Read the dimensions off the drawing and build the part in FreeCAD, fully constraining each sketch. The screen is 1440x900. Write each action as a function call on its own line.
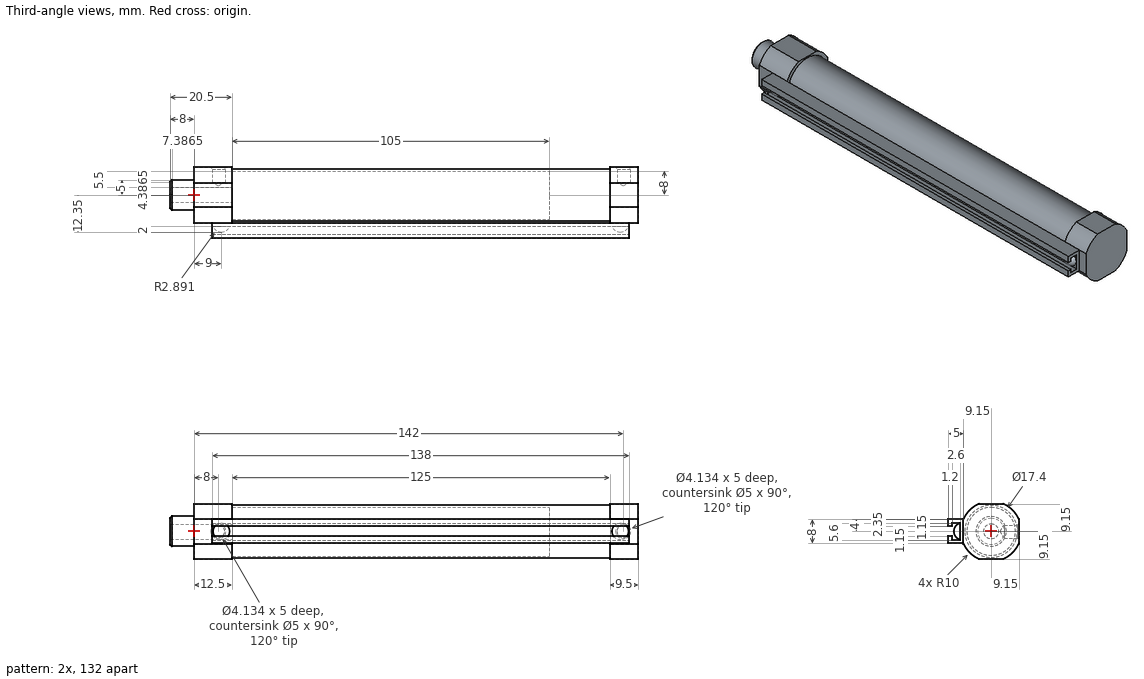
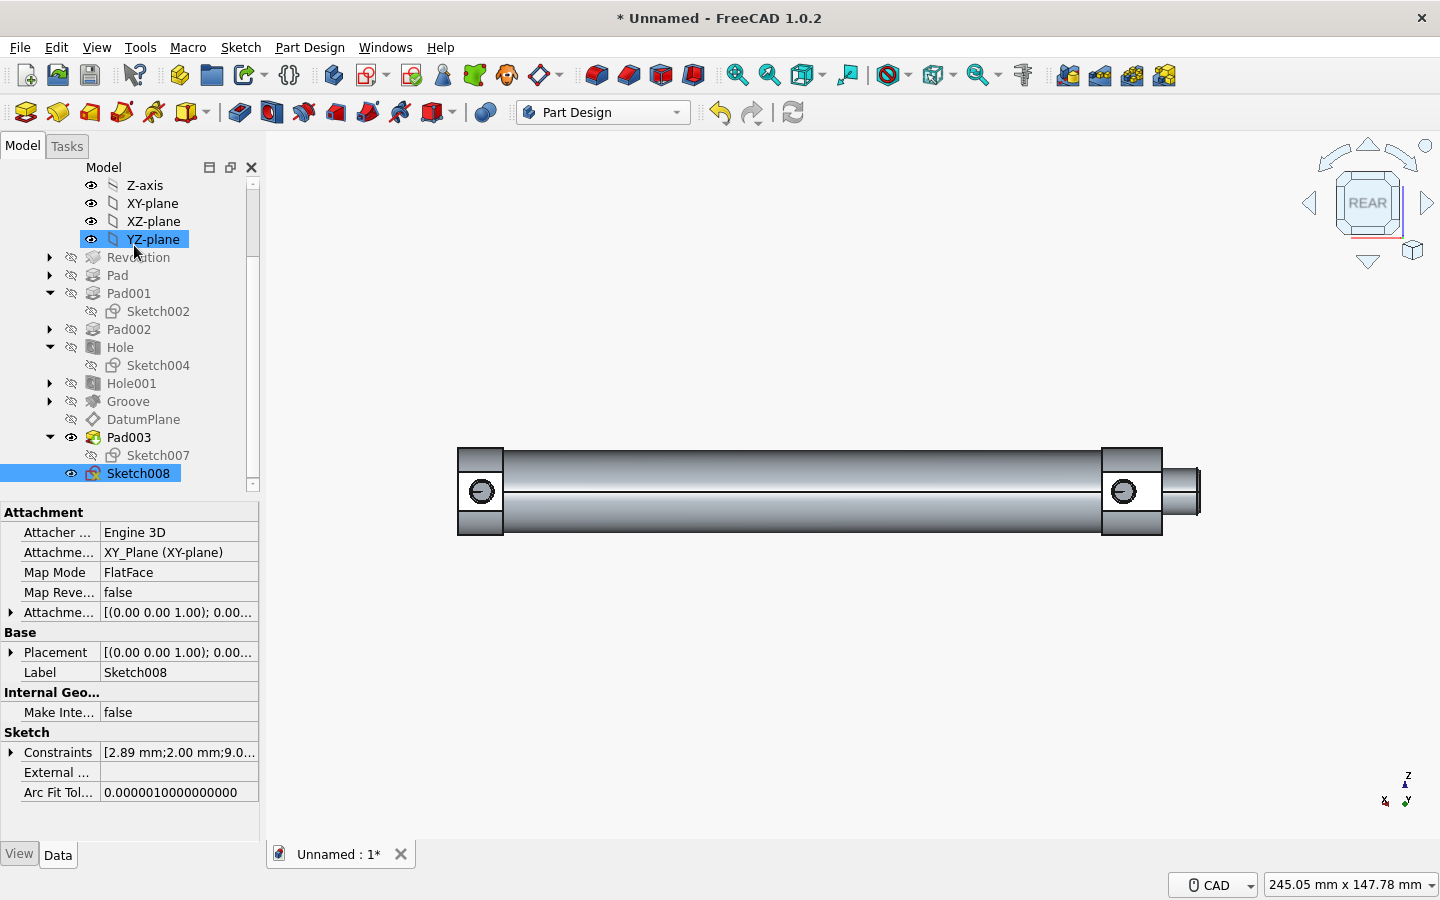
click(58, 112)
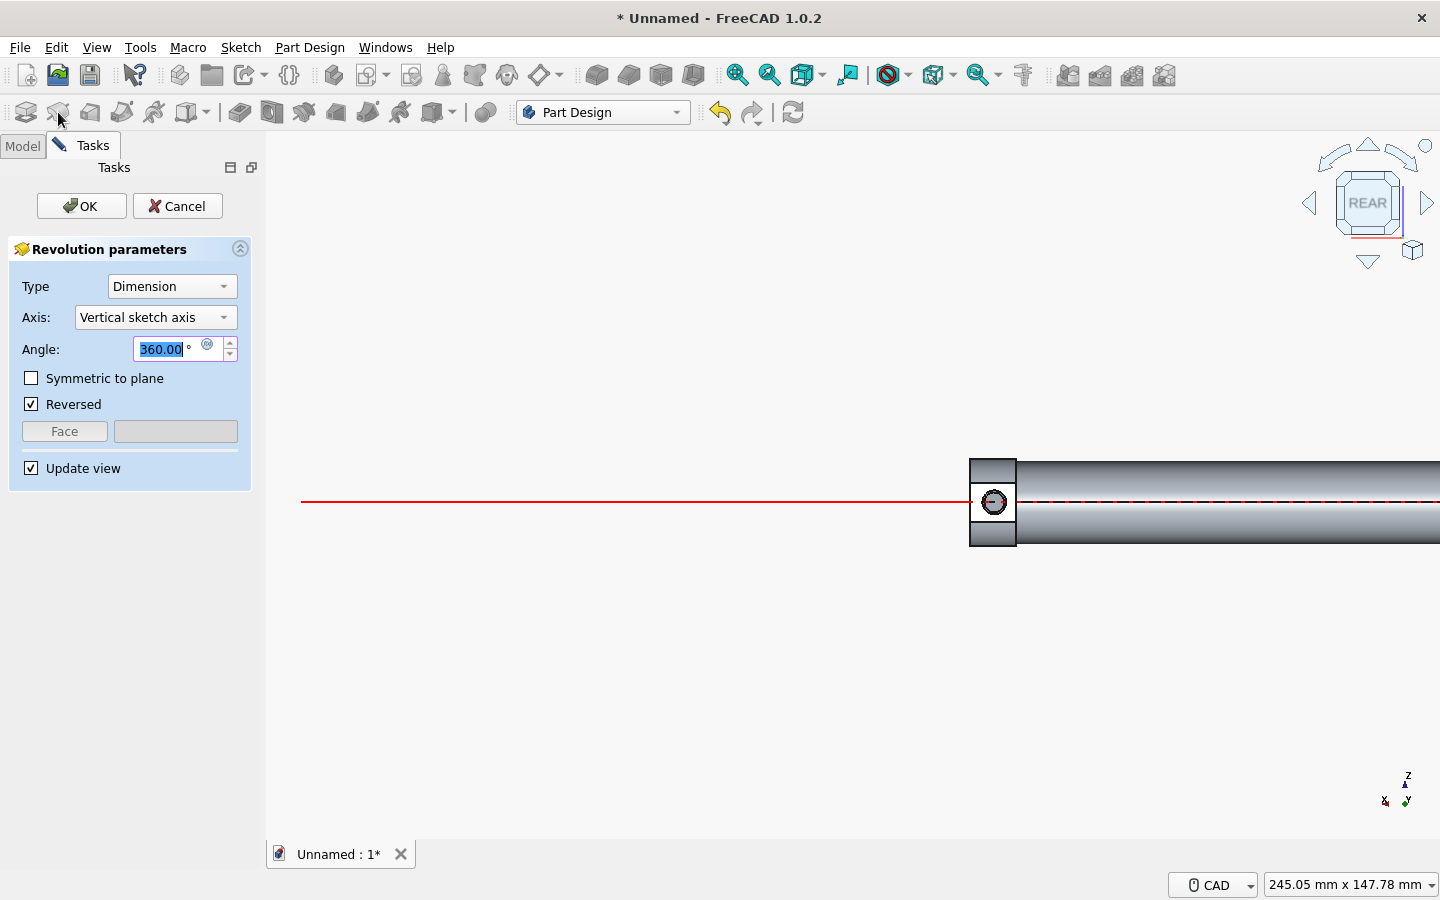
click(156, 318)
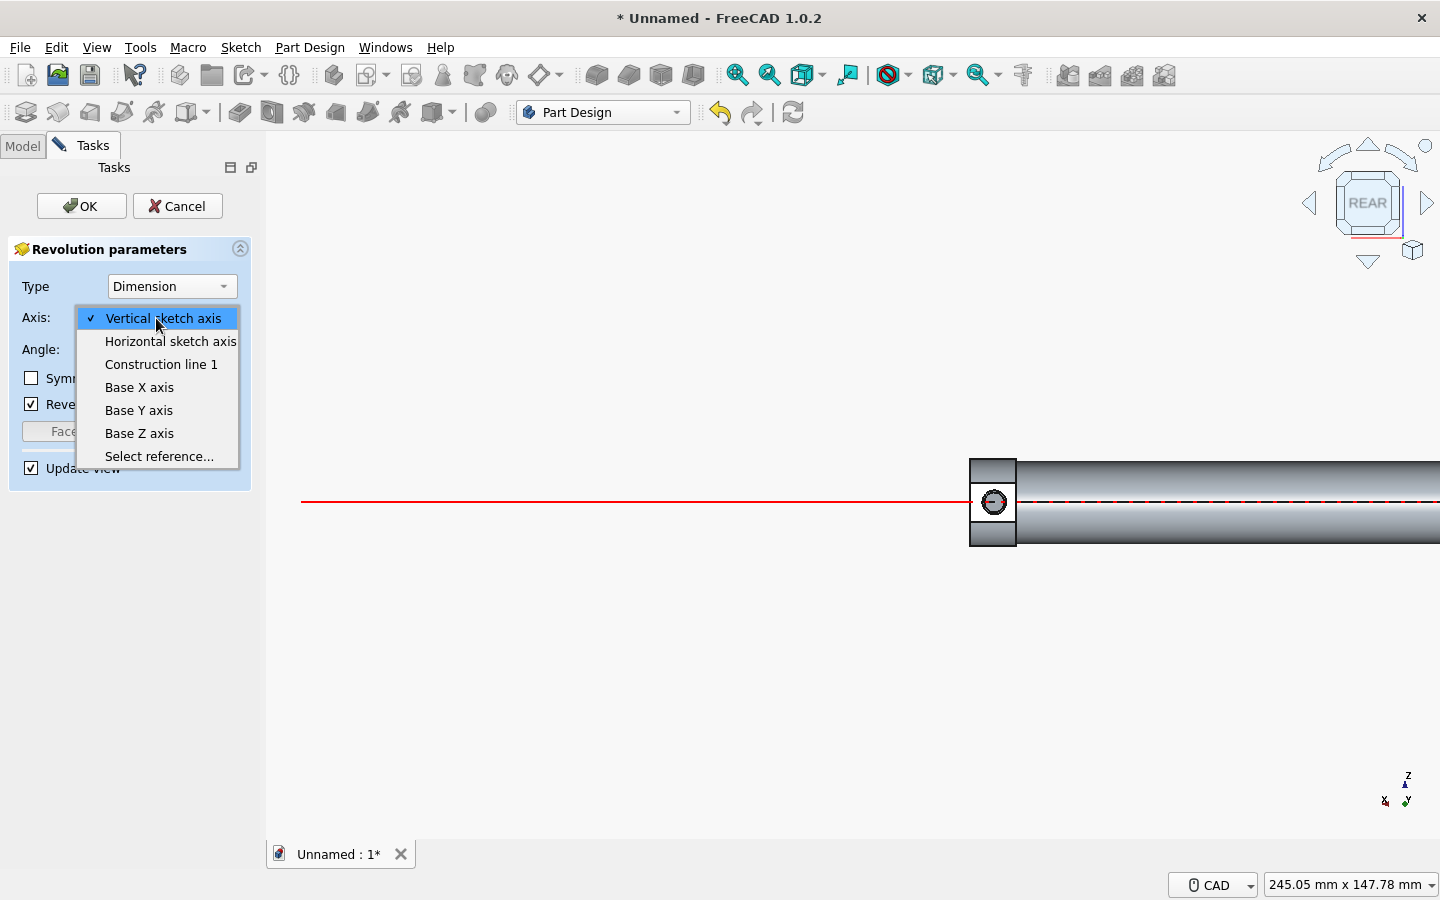
click(156, 364)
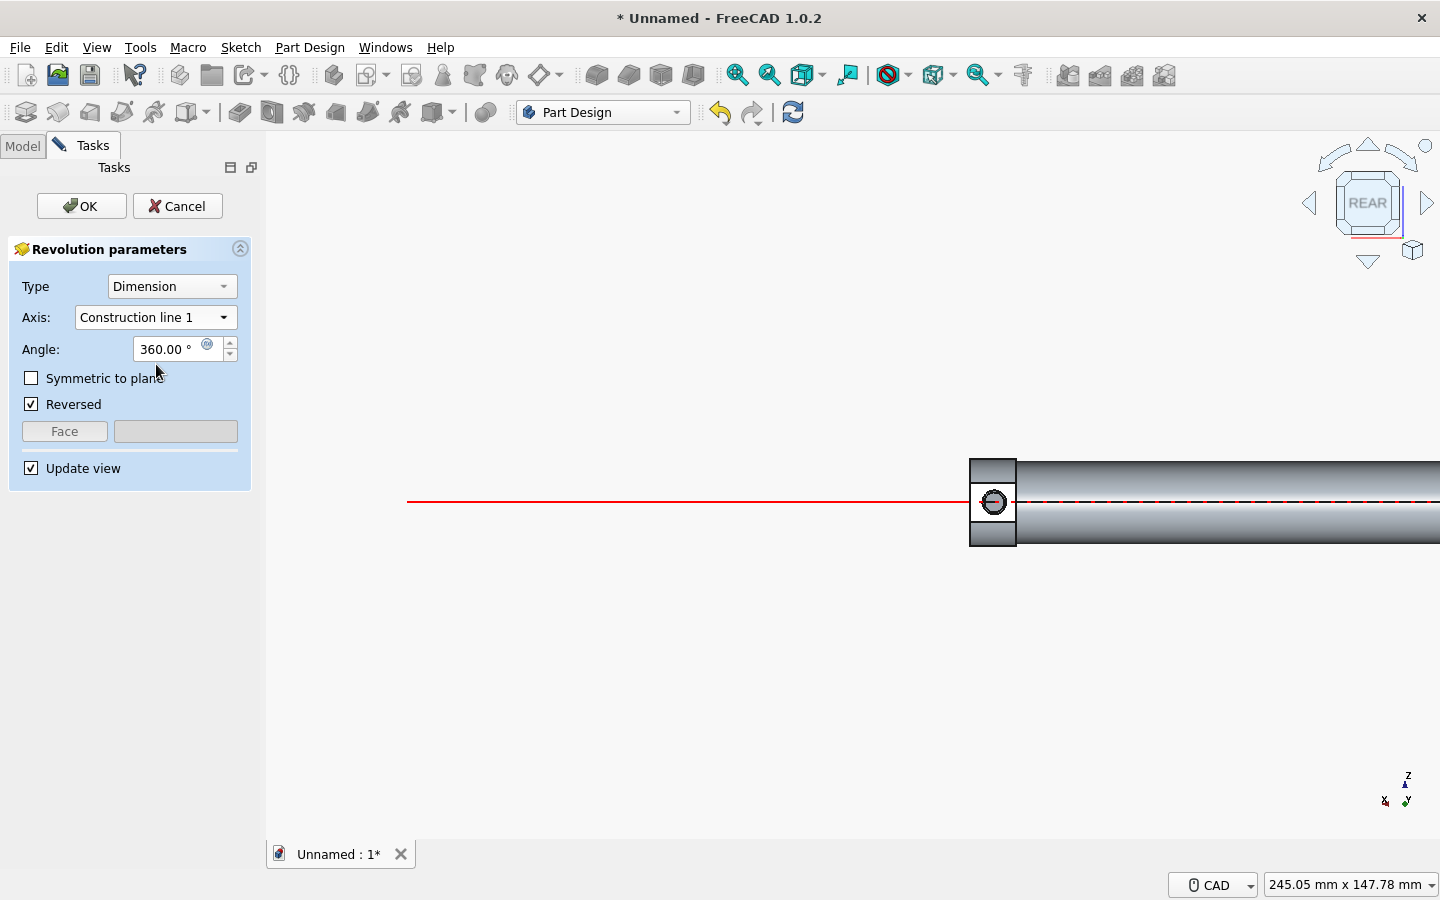
click(82, 206)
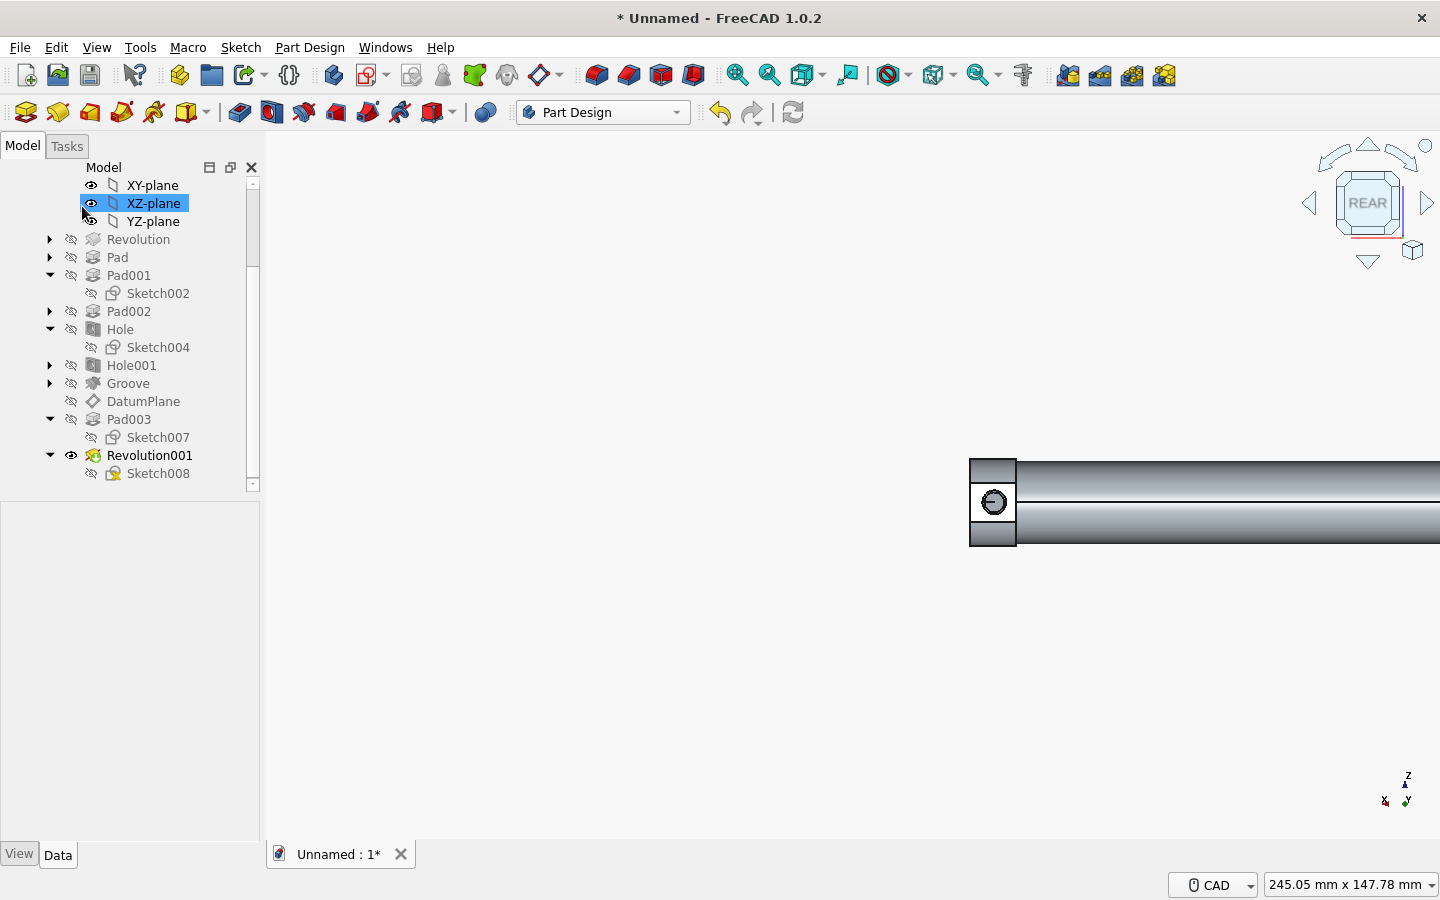
click(738, 76)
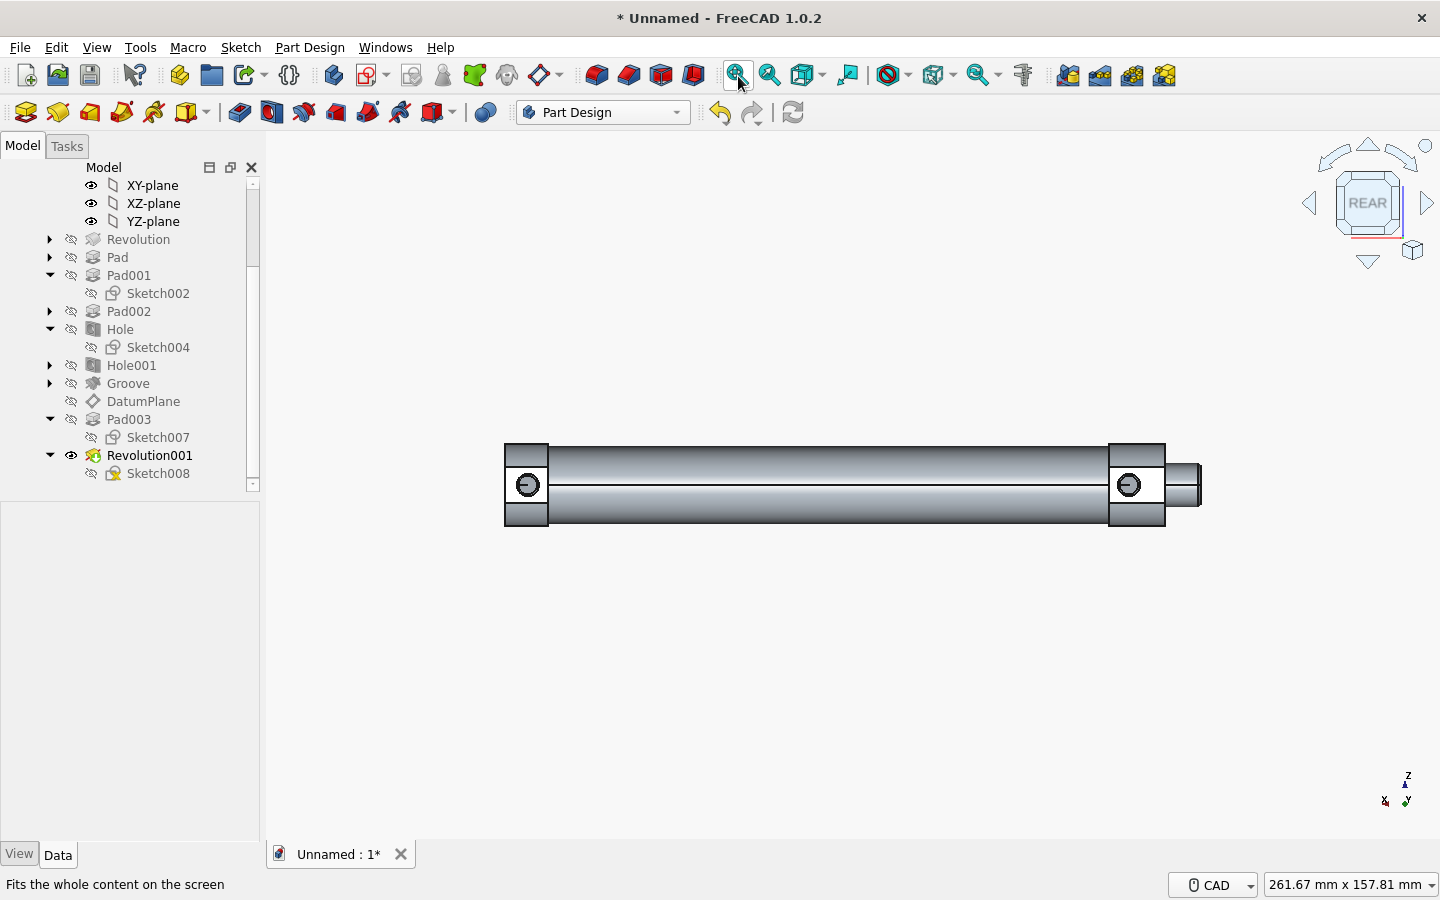
click(116, 455)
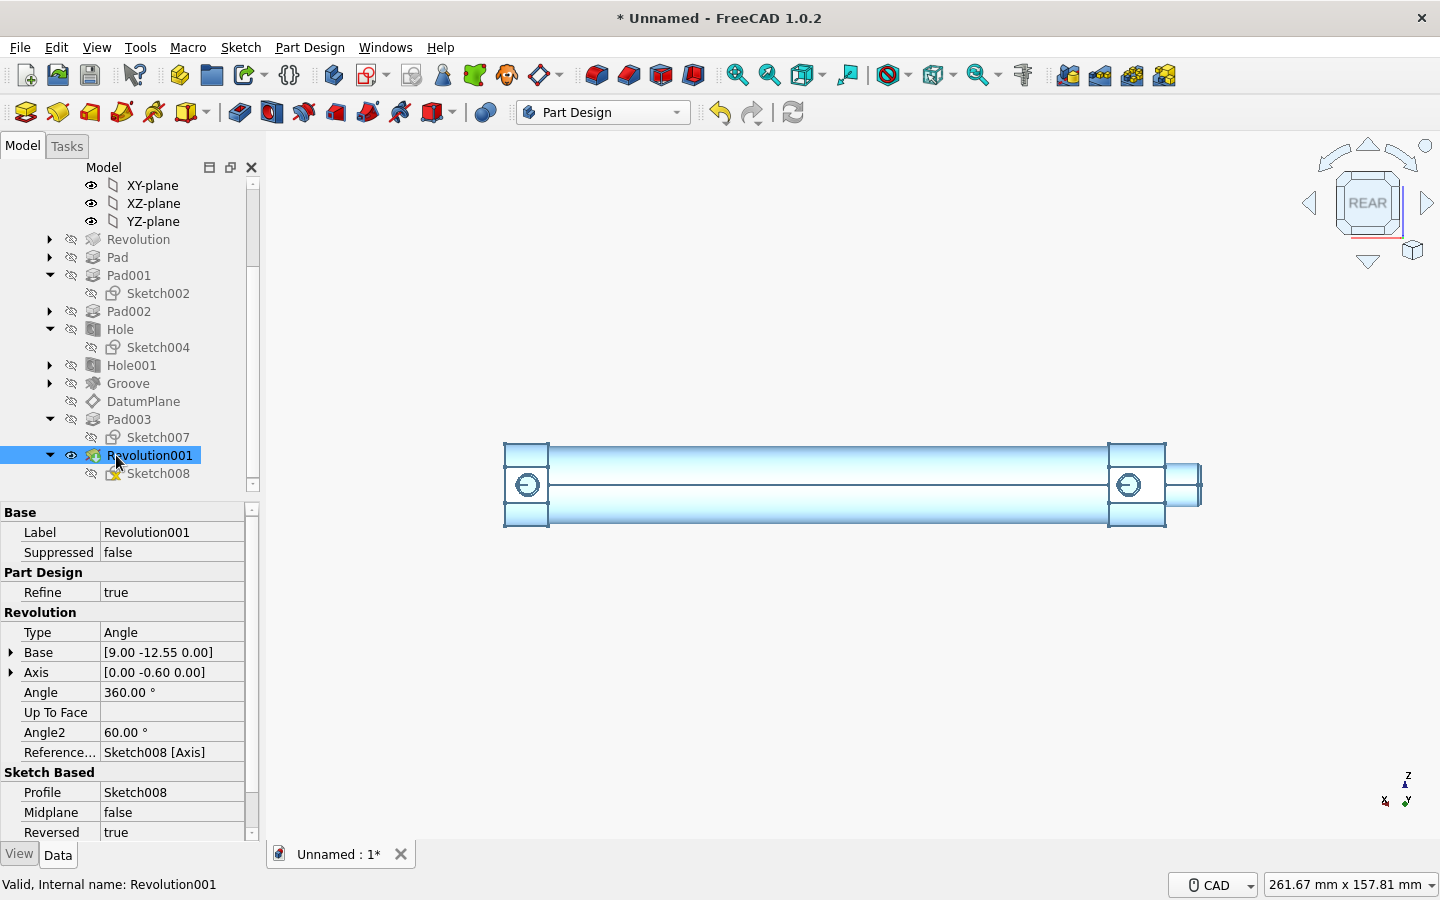
click(1100, 76)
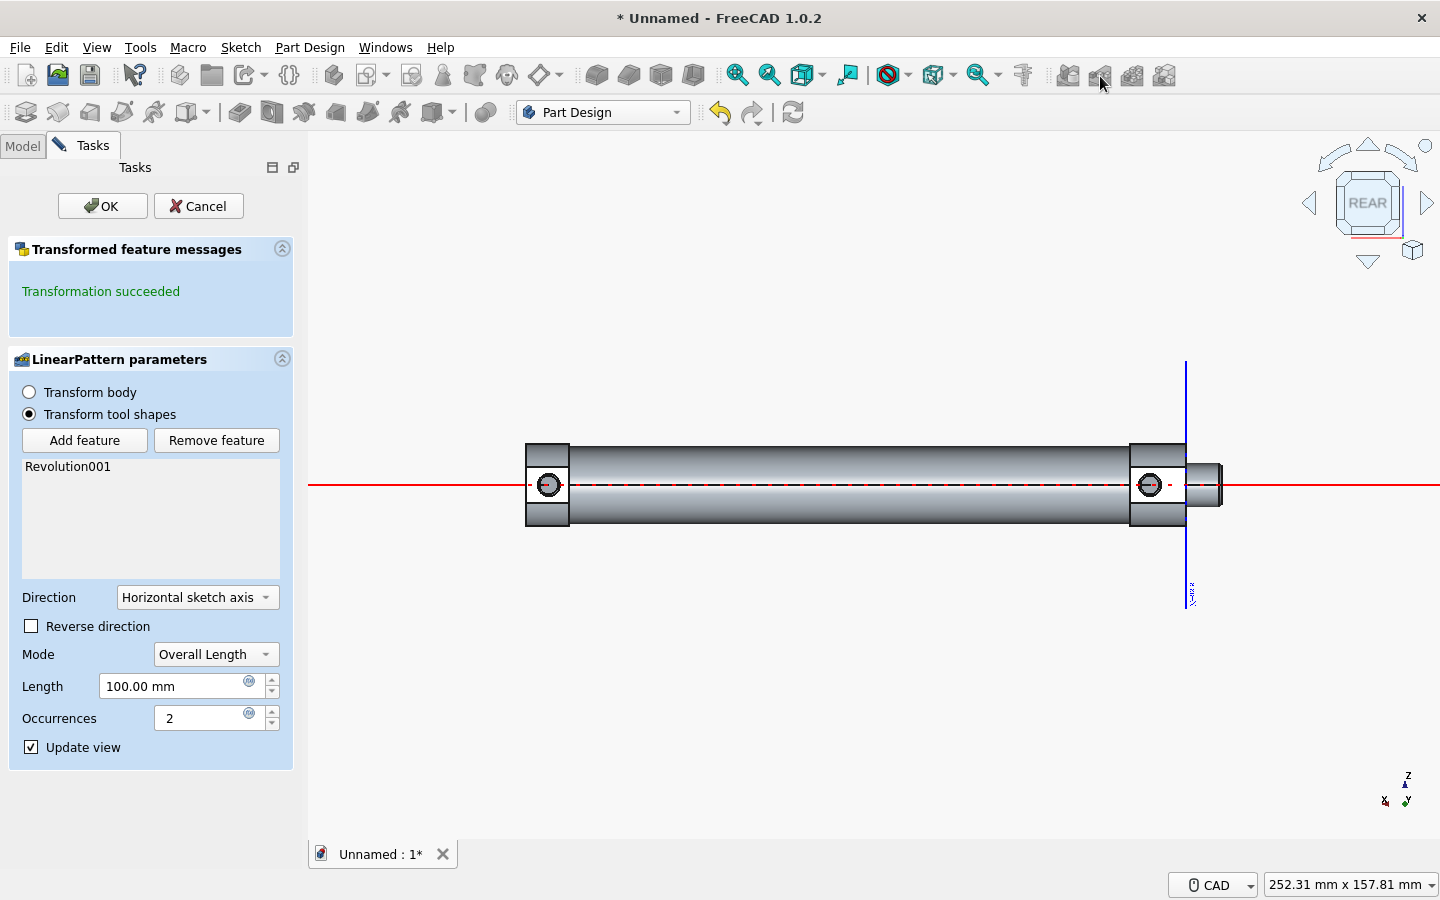
click(198, 598)